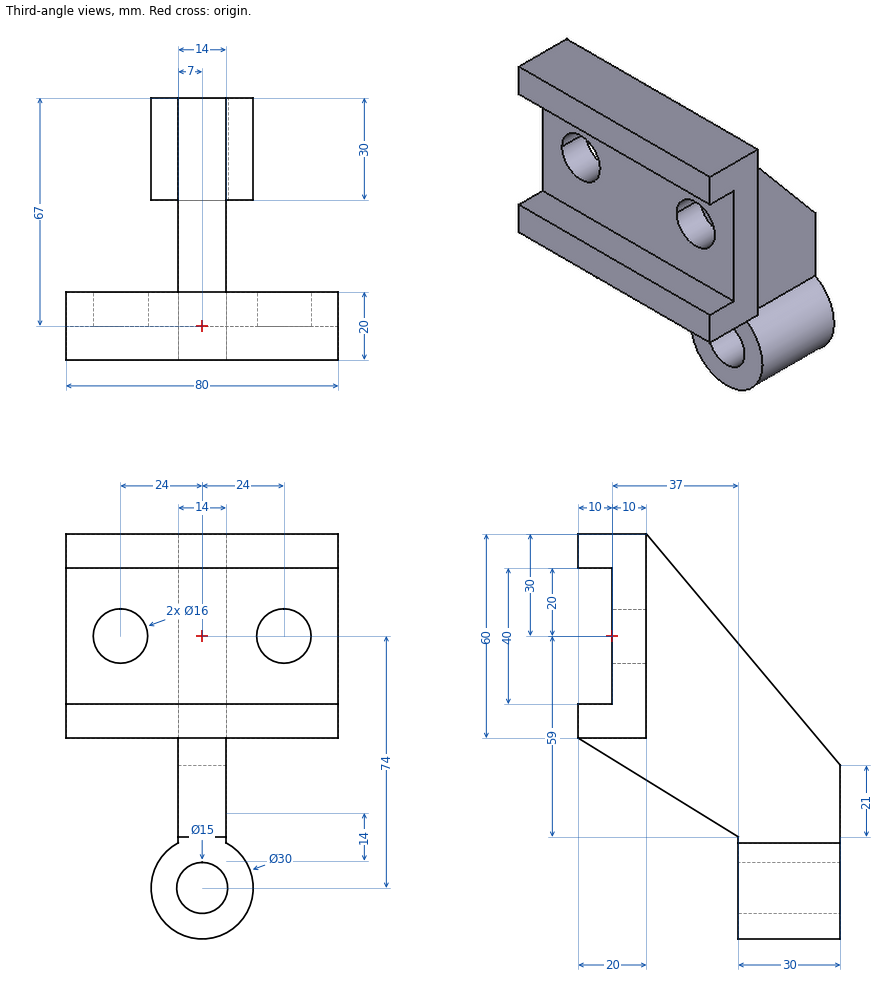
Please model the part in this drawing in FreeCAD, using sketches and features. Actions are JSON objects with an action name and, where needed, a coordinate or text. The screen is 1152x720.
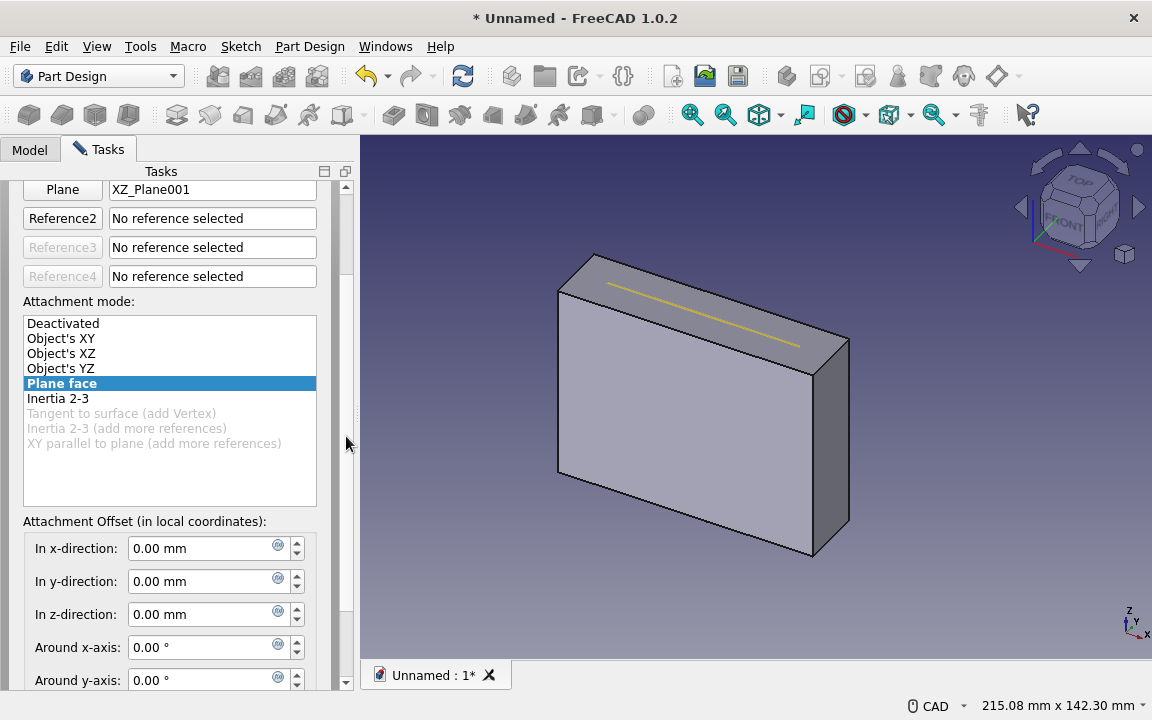
{"action": "triple_click", "coordinate": [210, 614]}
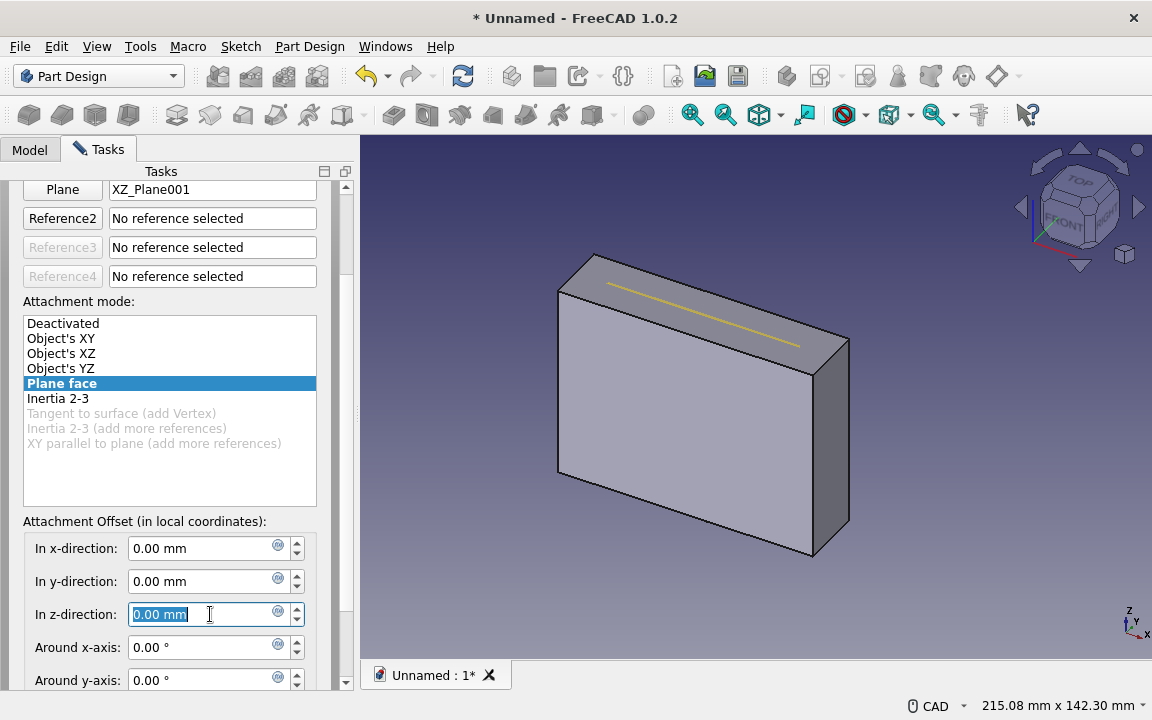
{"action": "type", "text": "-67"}
{"action": "key", "text": "Tab"}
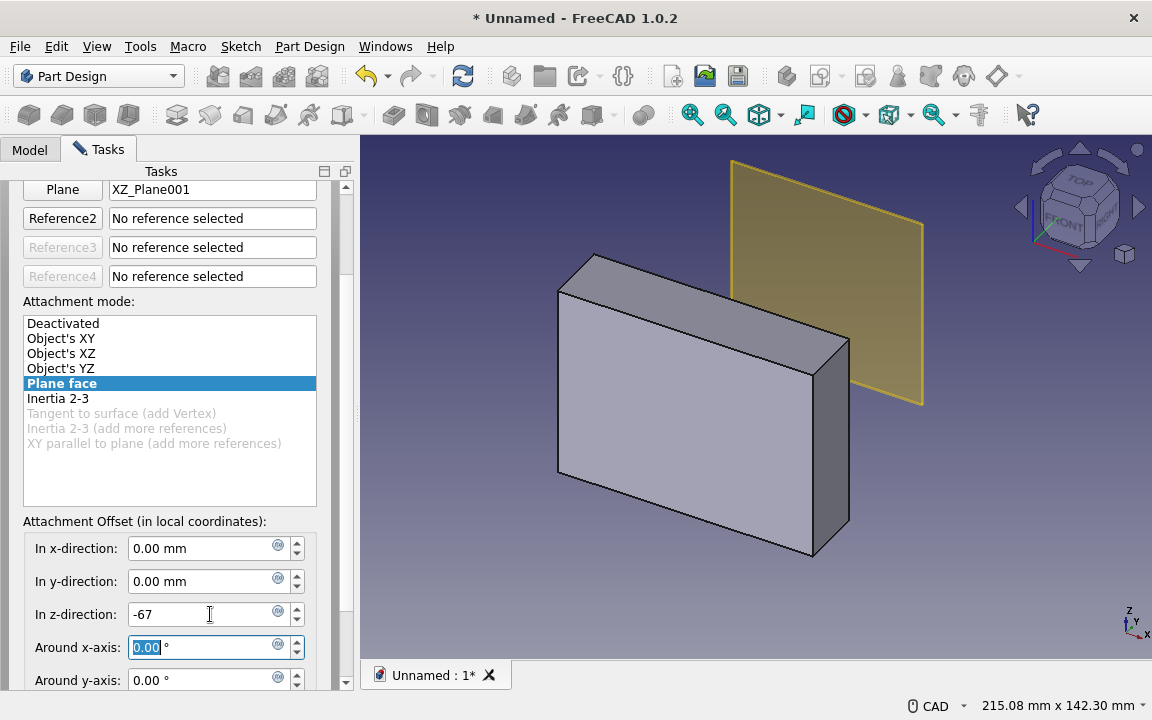
{"action": "scroll", "coordinate": [346, 436], "scroll_direction": "up", "scroll_amount": 3}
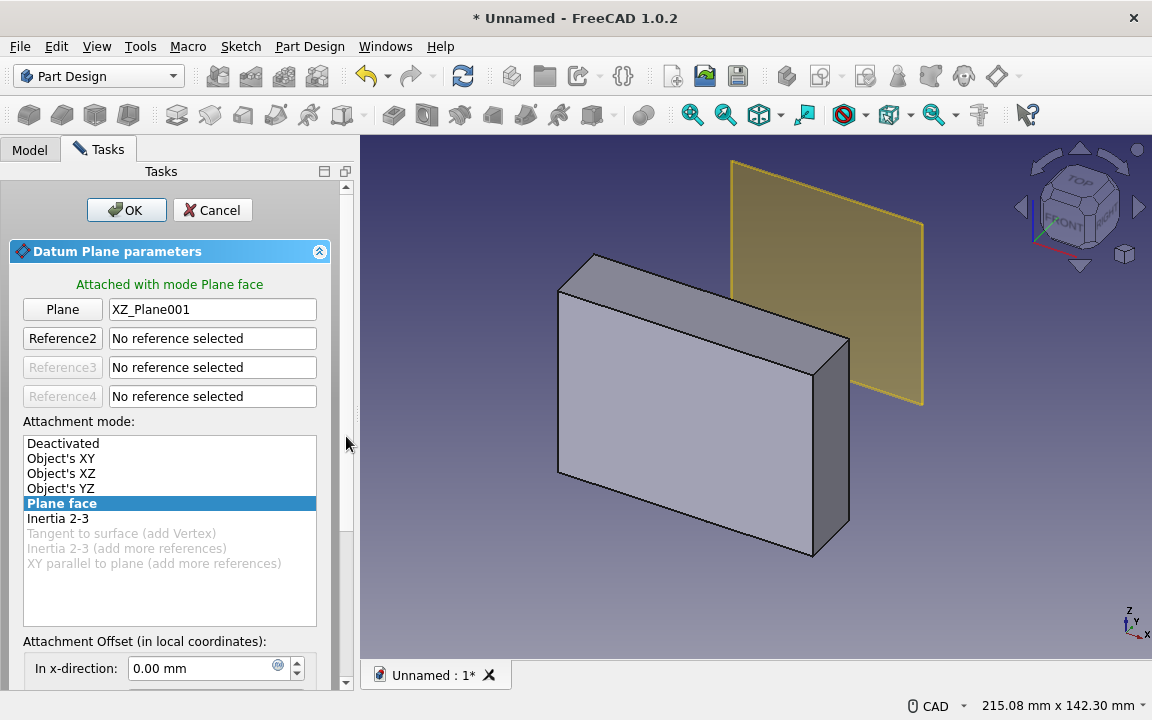
{"action": "left_click", "coordinate": [127, 210]}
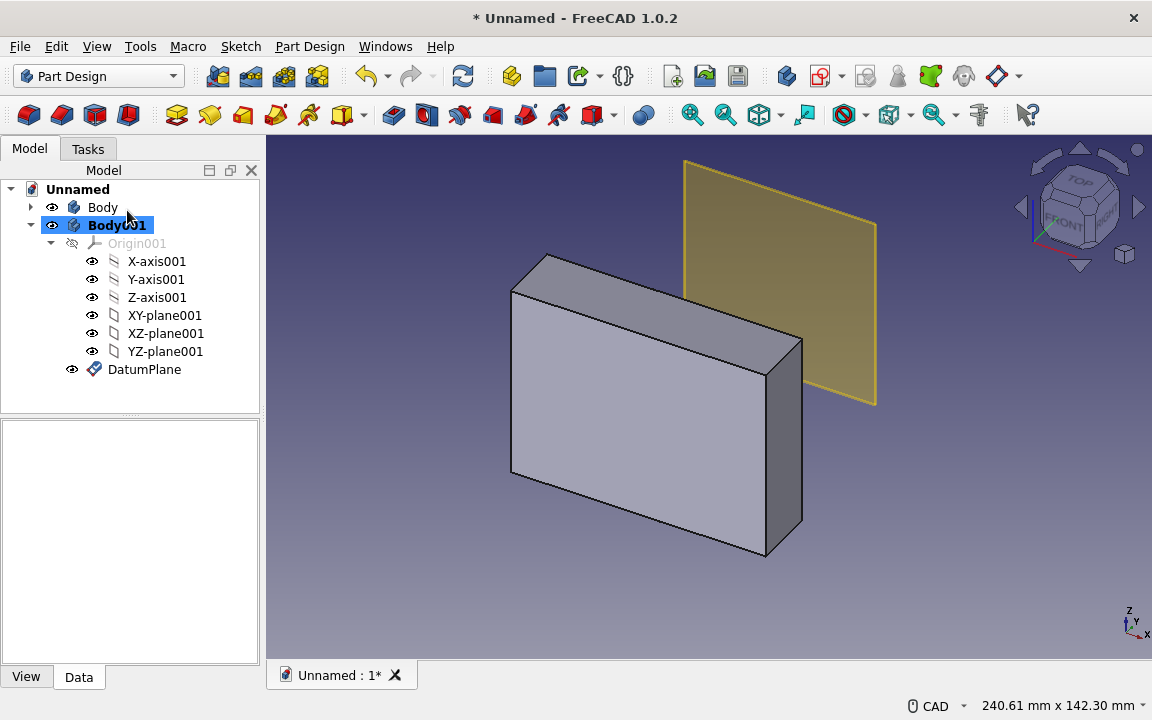
{"action": "left_click", "coordinate": [117, 369]}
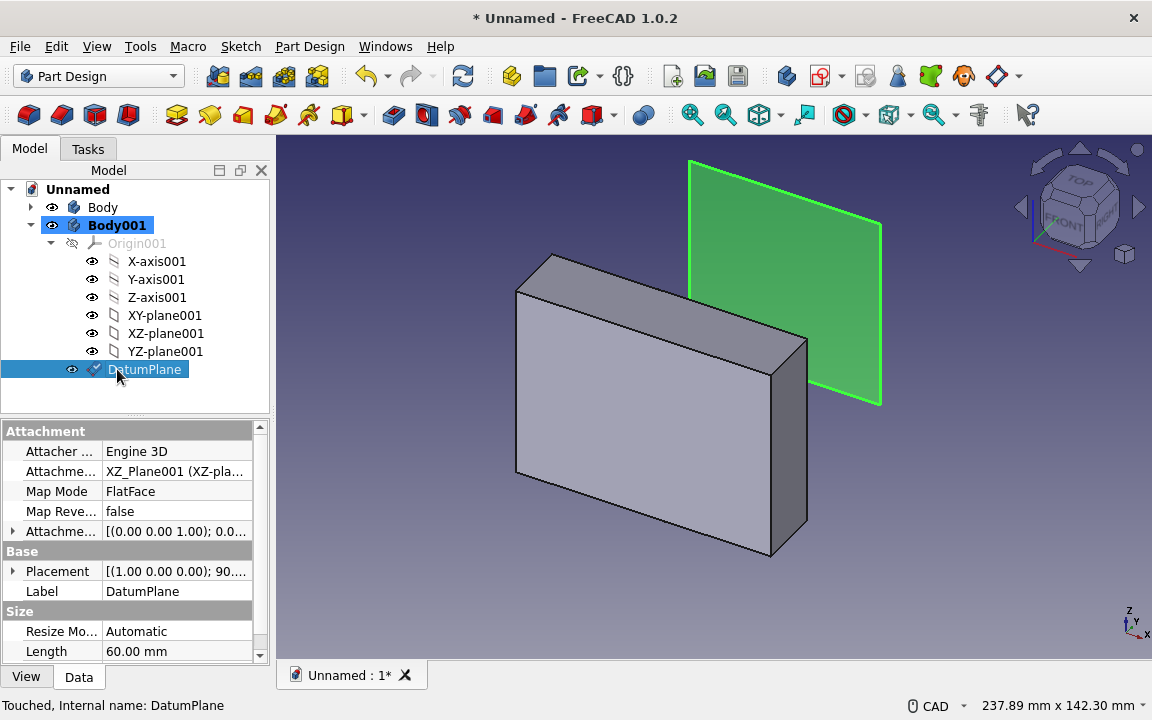
{"action": "left_click", "coordinate": [820, 76]}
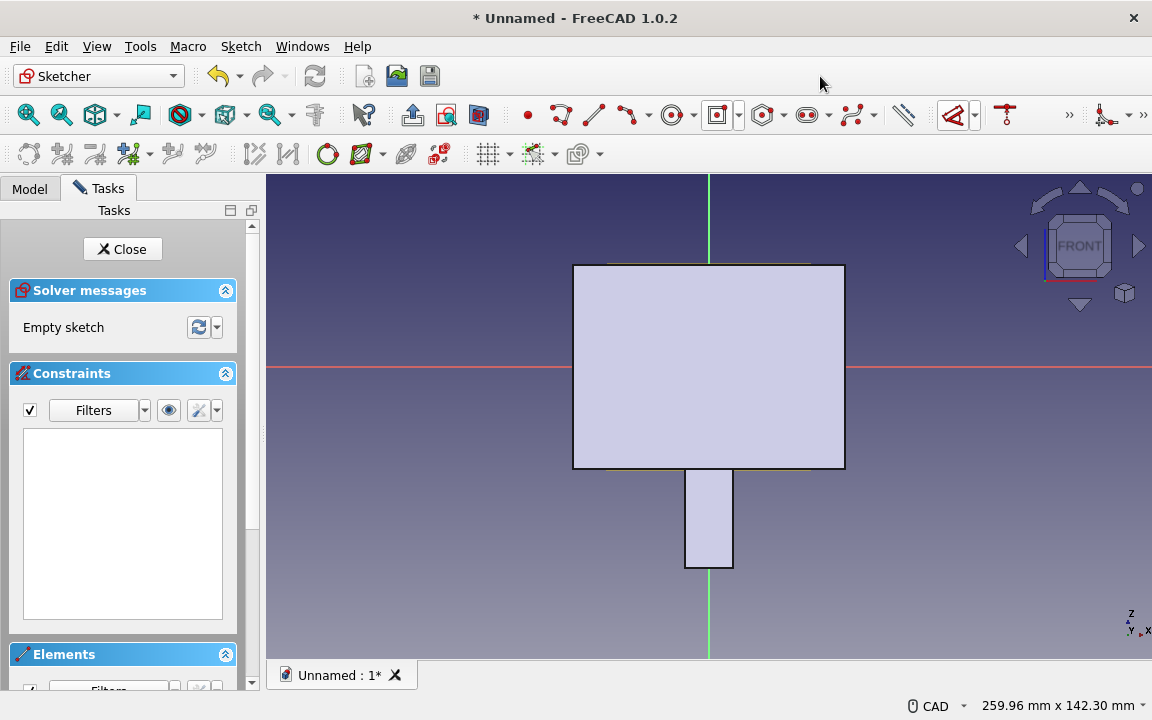
{"action": "scroll", "coordinate": [640, 416], "scroll_direction": "down", "scroll_amount": 5}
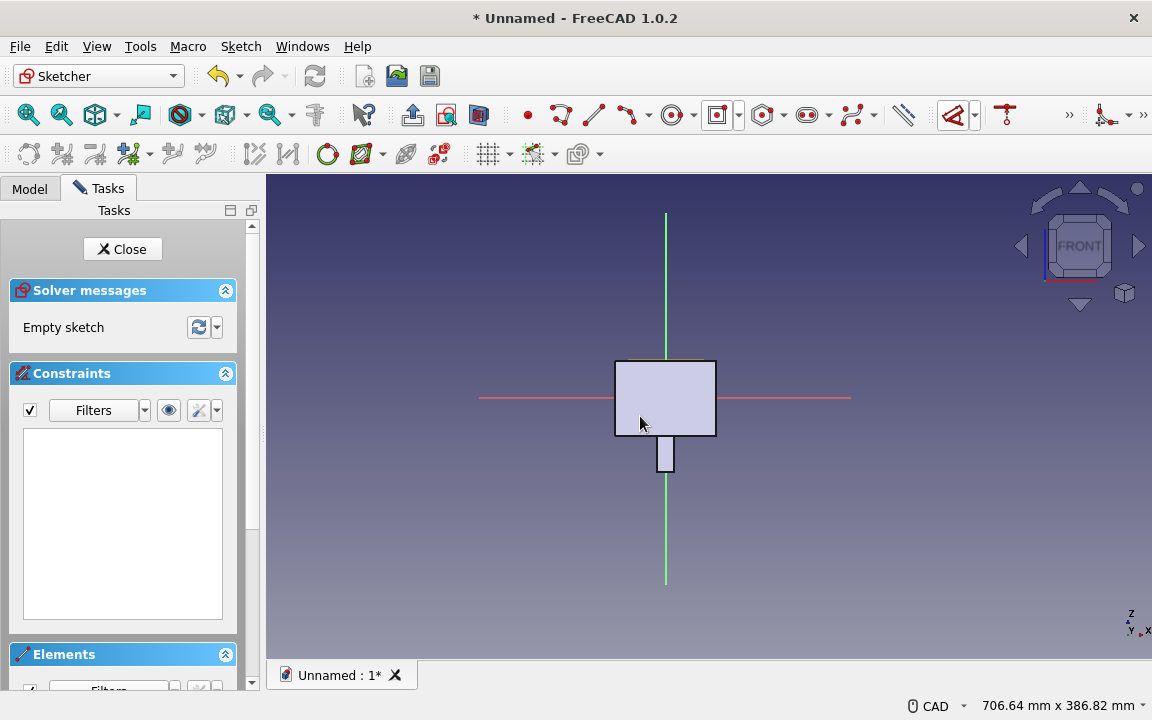
{"action": "scroll", "coordinate": [670, 503], "scroll_direction": "up", "scroll_amount": 10}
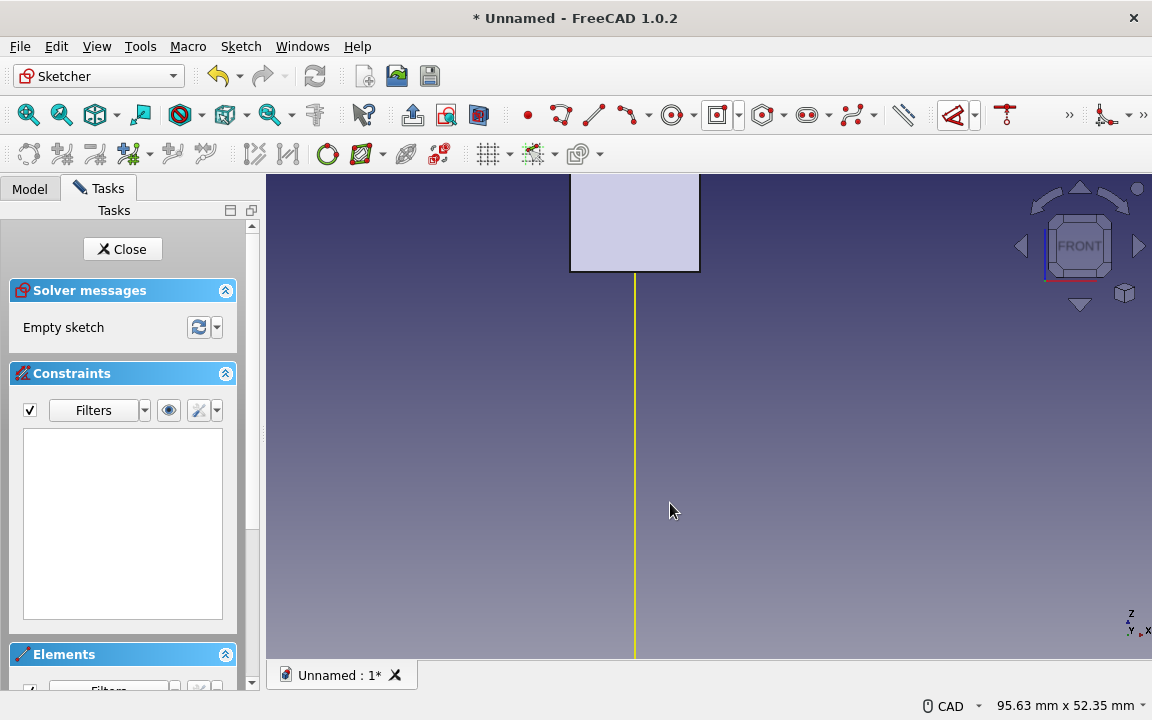
{"action": "left_click", "coordinate": [672, 116]}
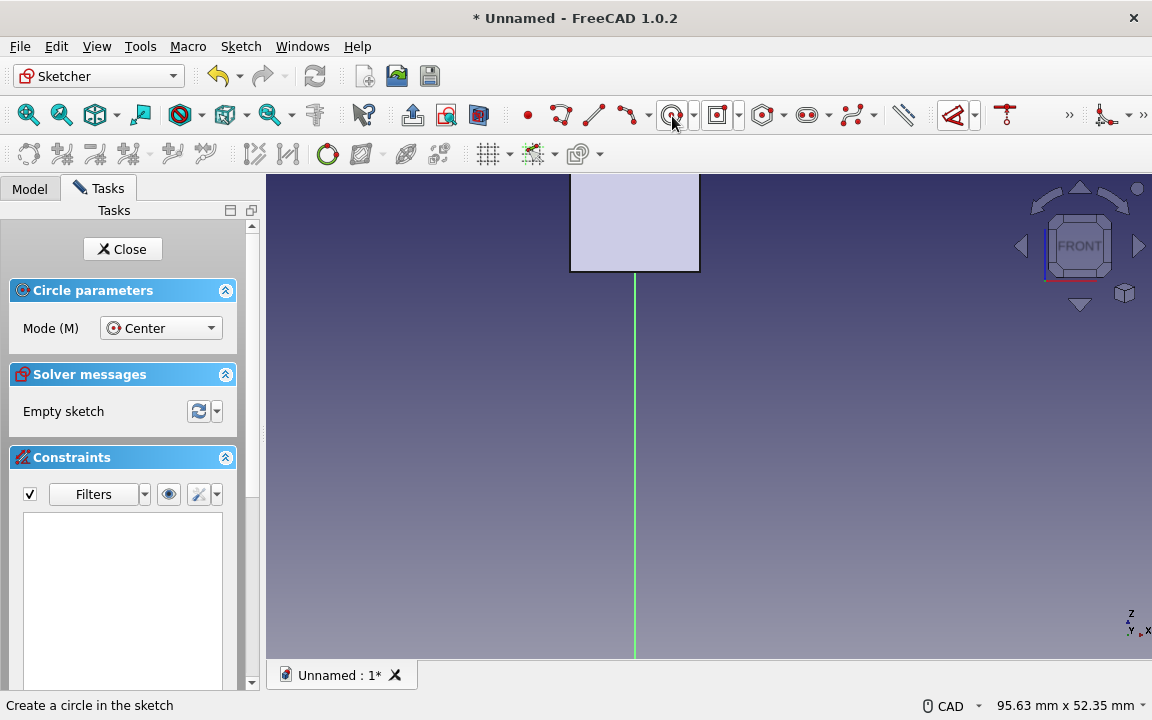
{"action": "left_click", "coordinate": [635, 411]}
{"action": "mouse_move", "coordinate": [733, 312]}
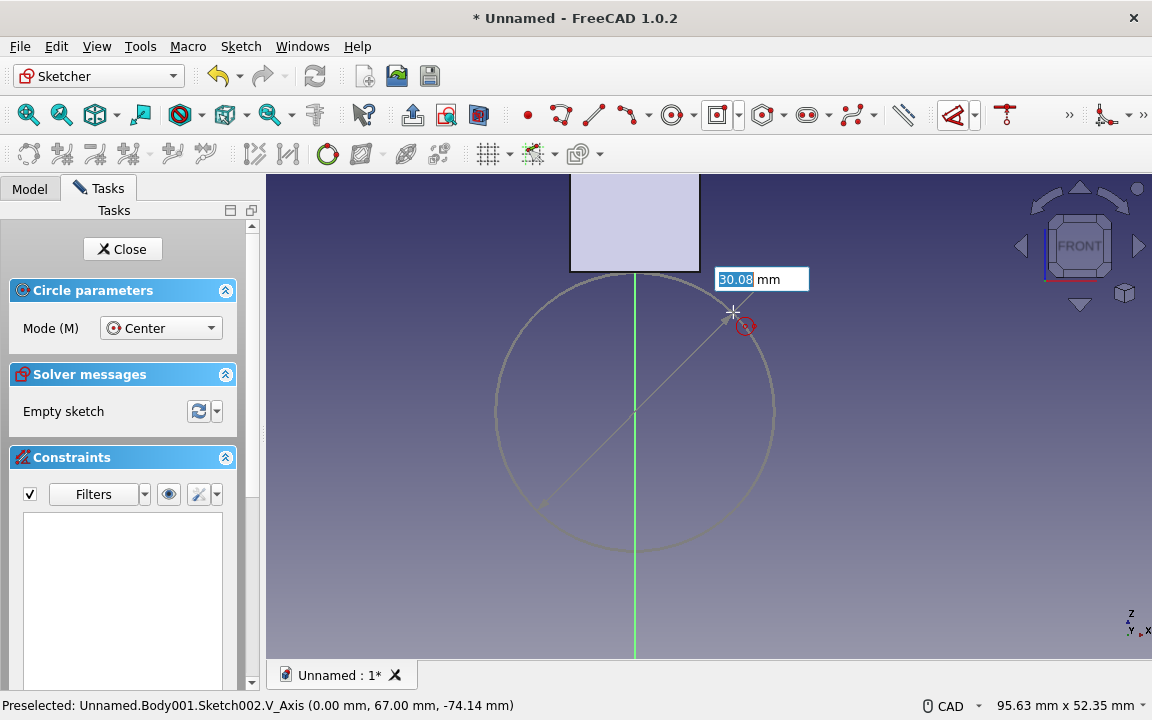
{"action": "type", "text": "30"}
{"action": "key", "text": "Return"}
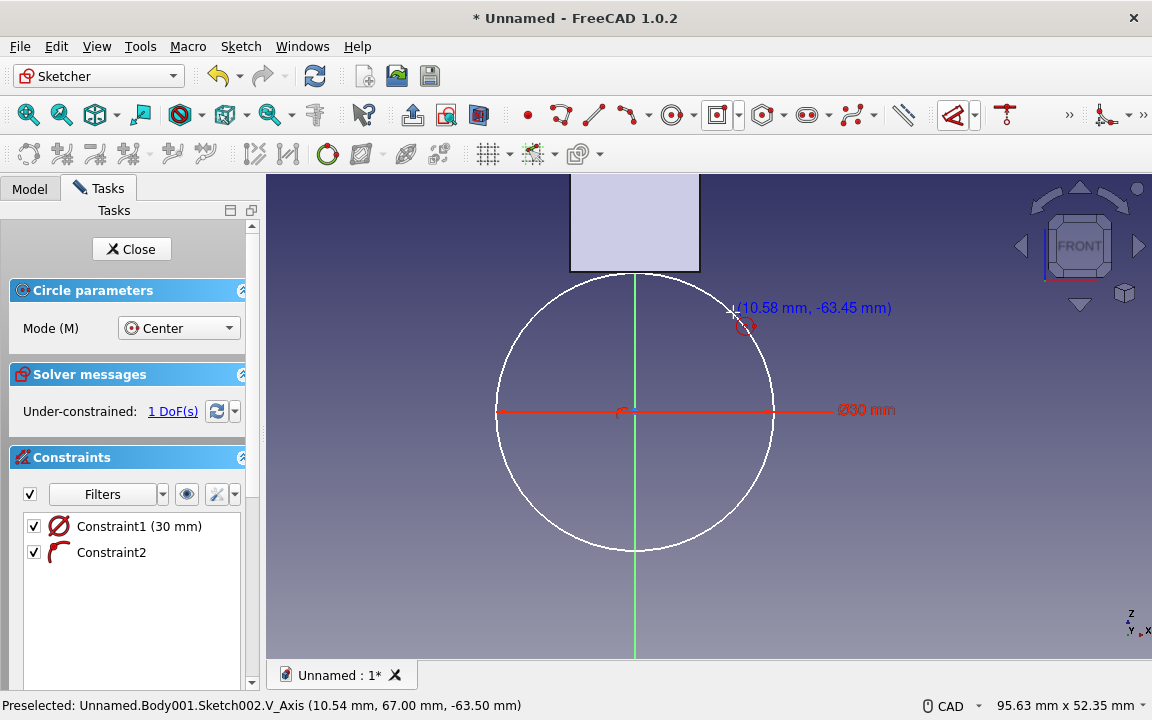
{"action": "left_click", "coordinate": [635, 412]}
{"action": "mouse_move", "coordinate": [684, 362]}